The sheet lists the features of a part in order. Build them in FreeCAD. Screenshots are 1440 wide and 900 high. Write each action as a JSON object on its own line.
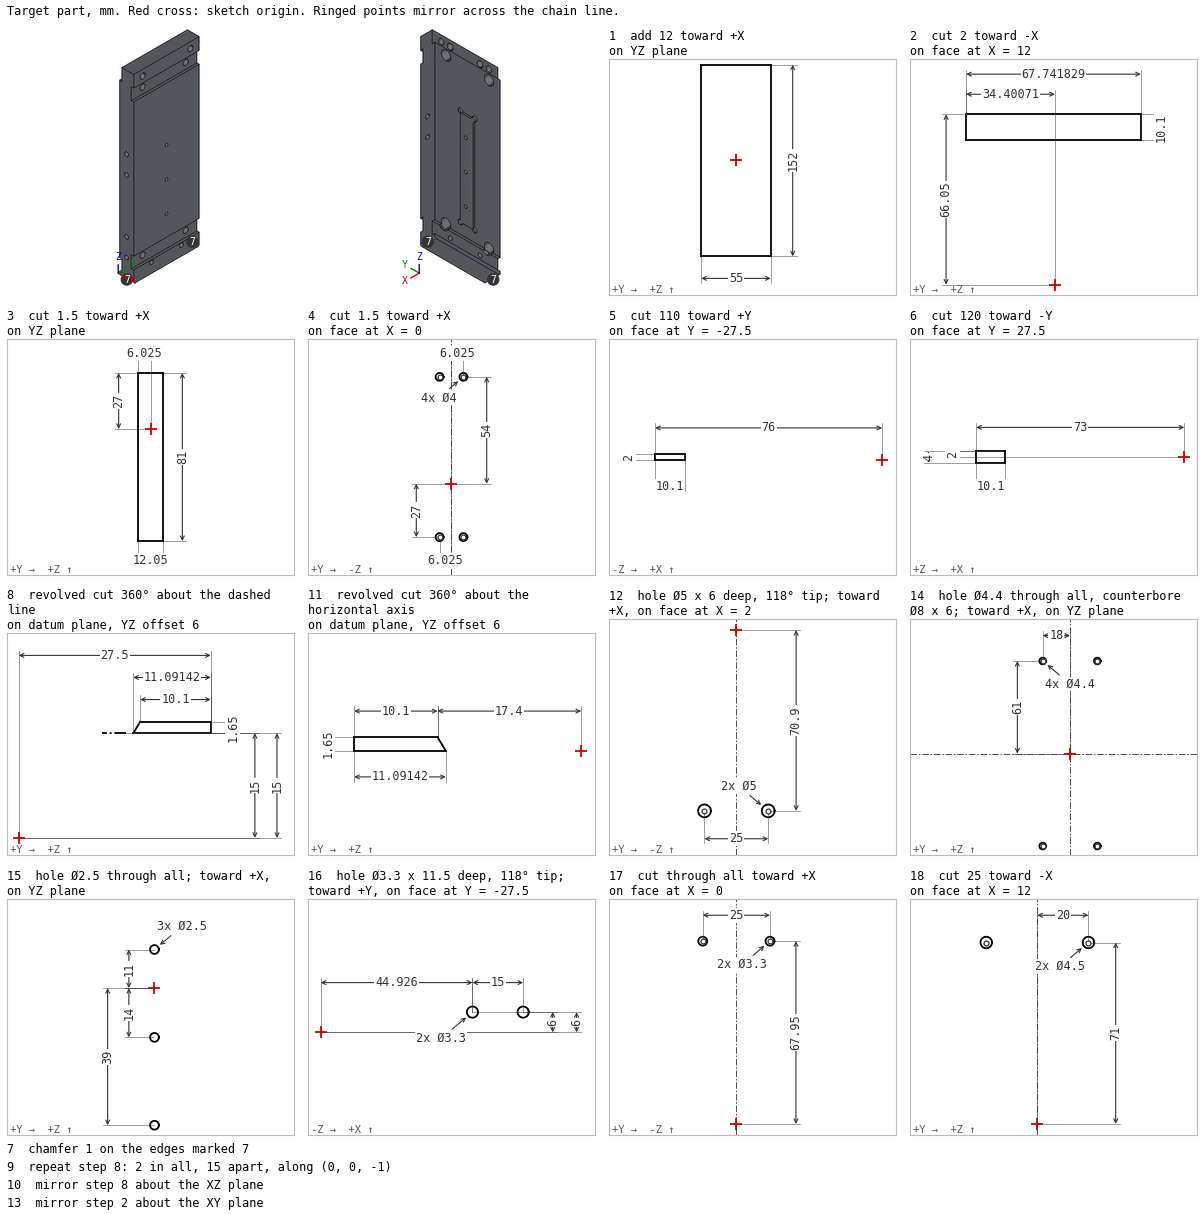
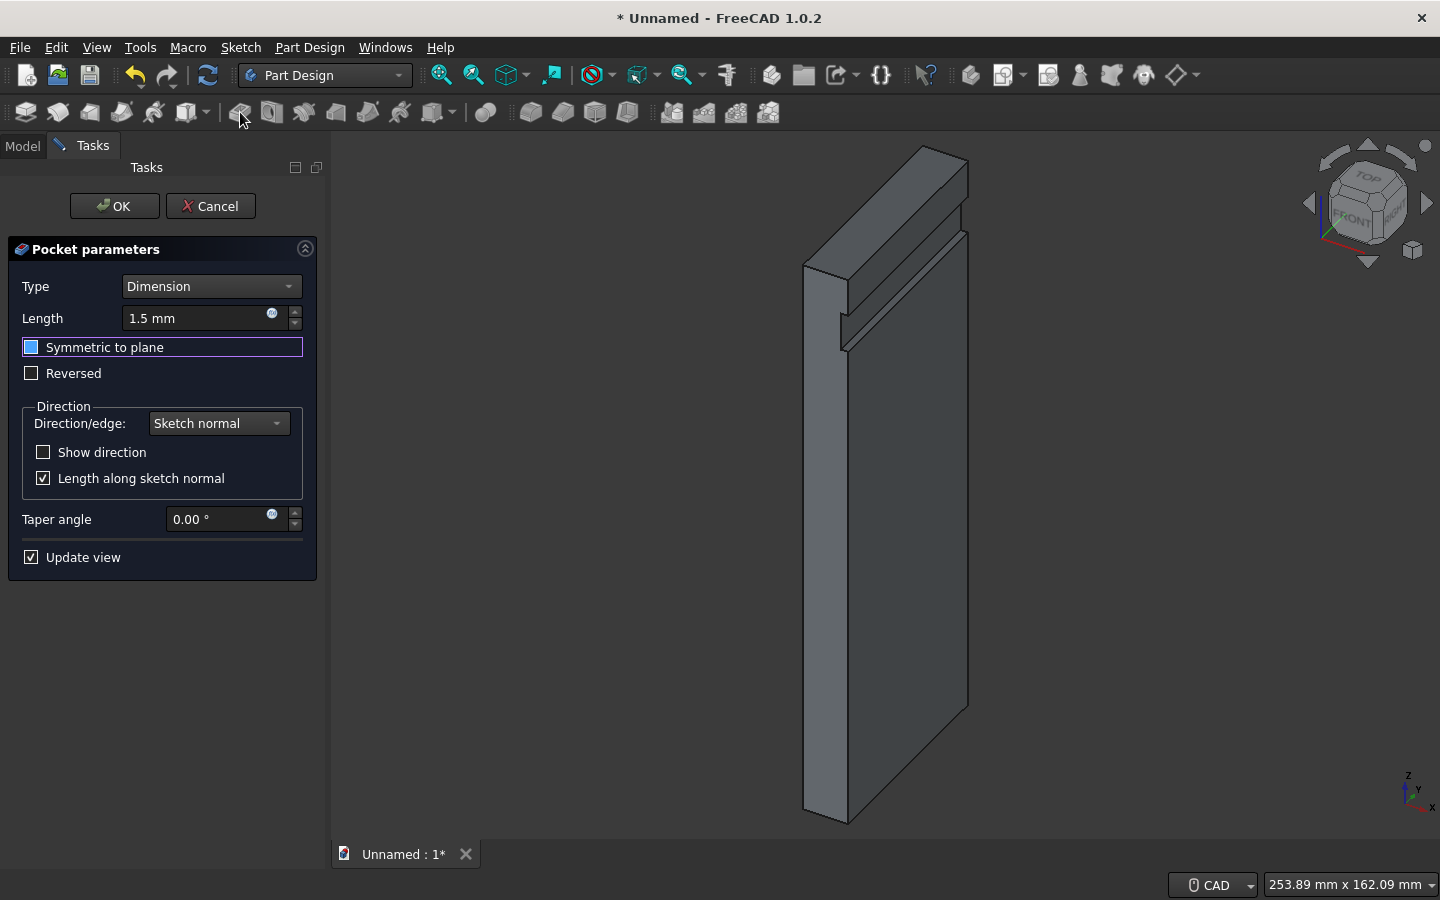
{"action": "left_click", "coordinate": [30, 373]}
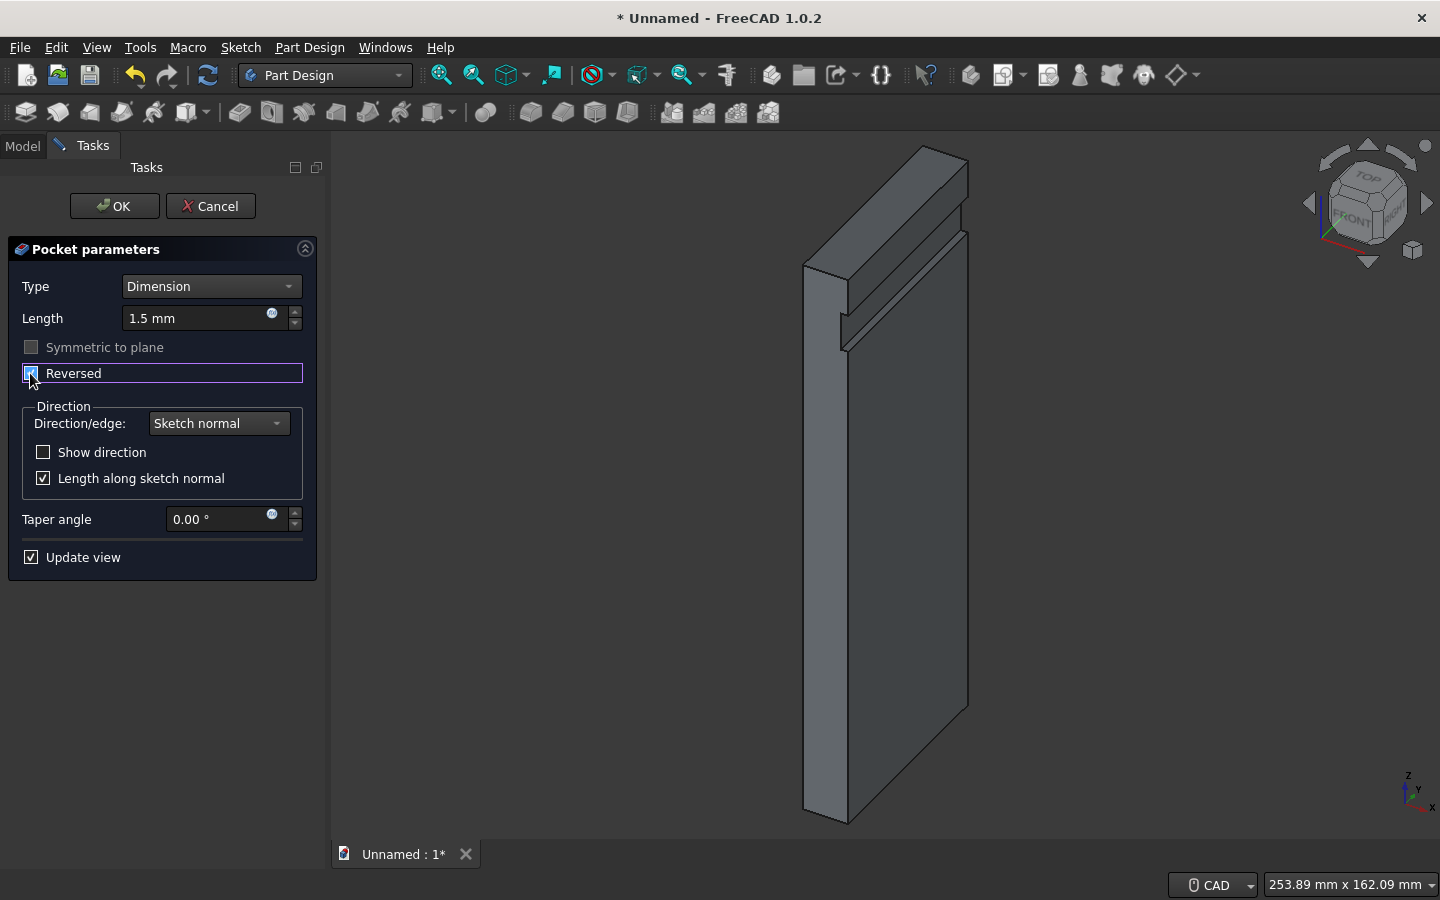
{"action": "left_click", "coordinate": [115, 206]}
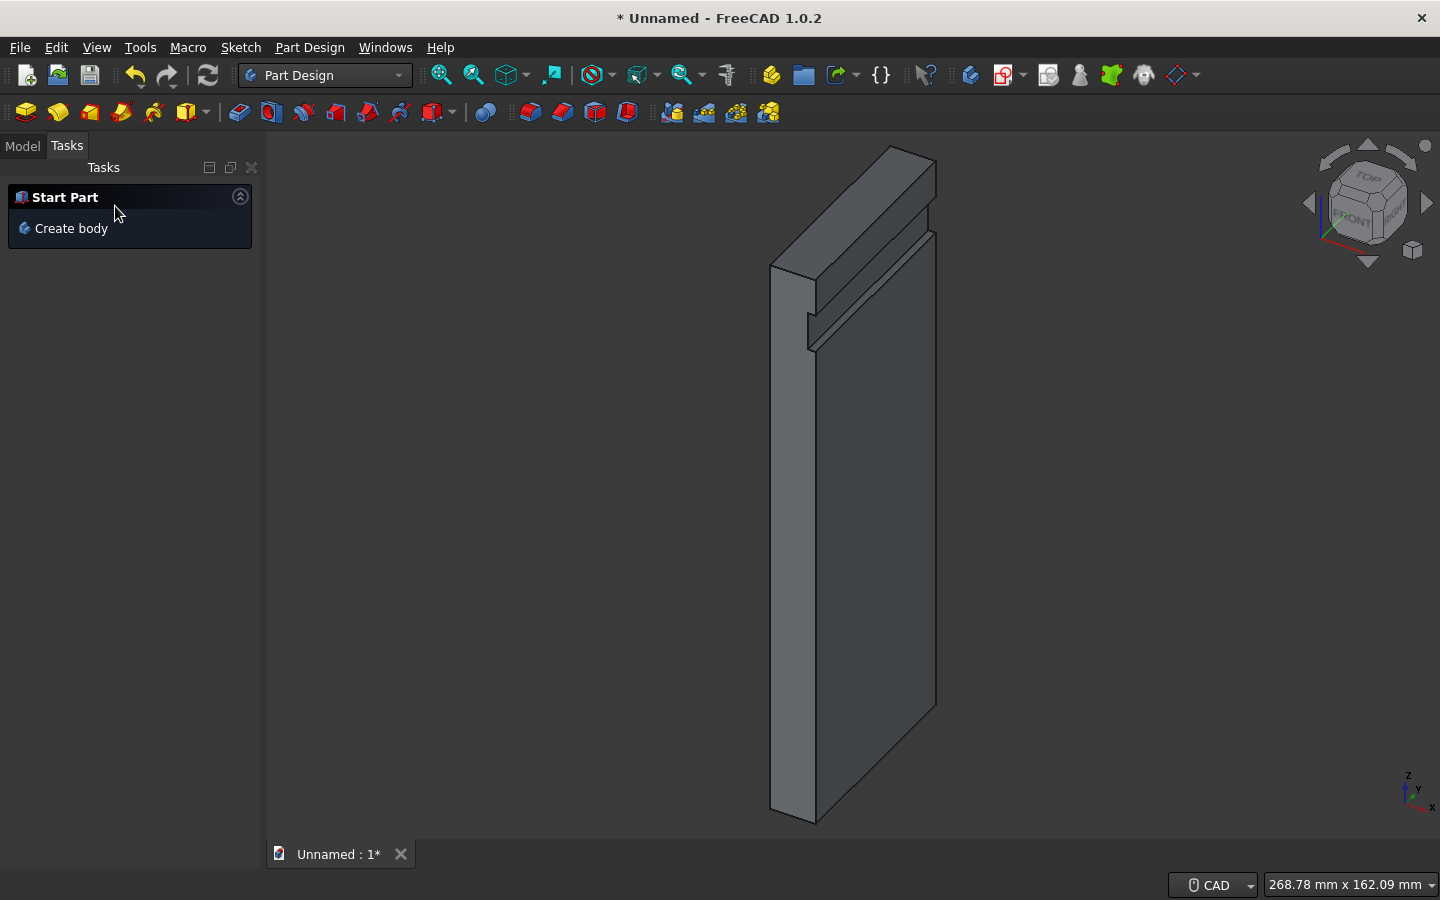
{"action": "key", "text": "6"}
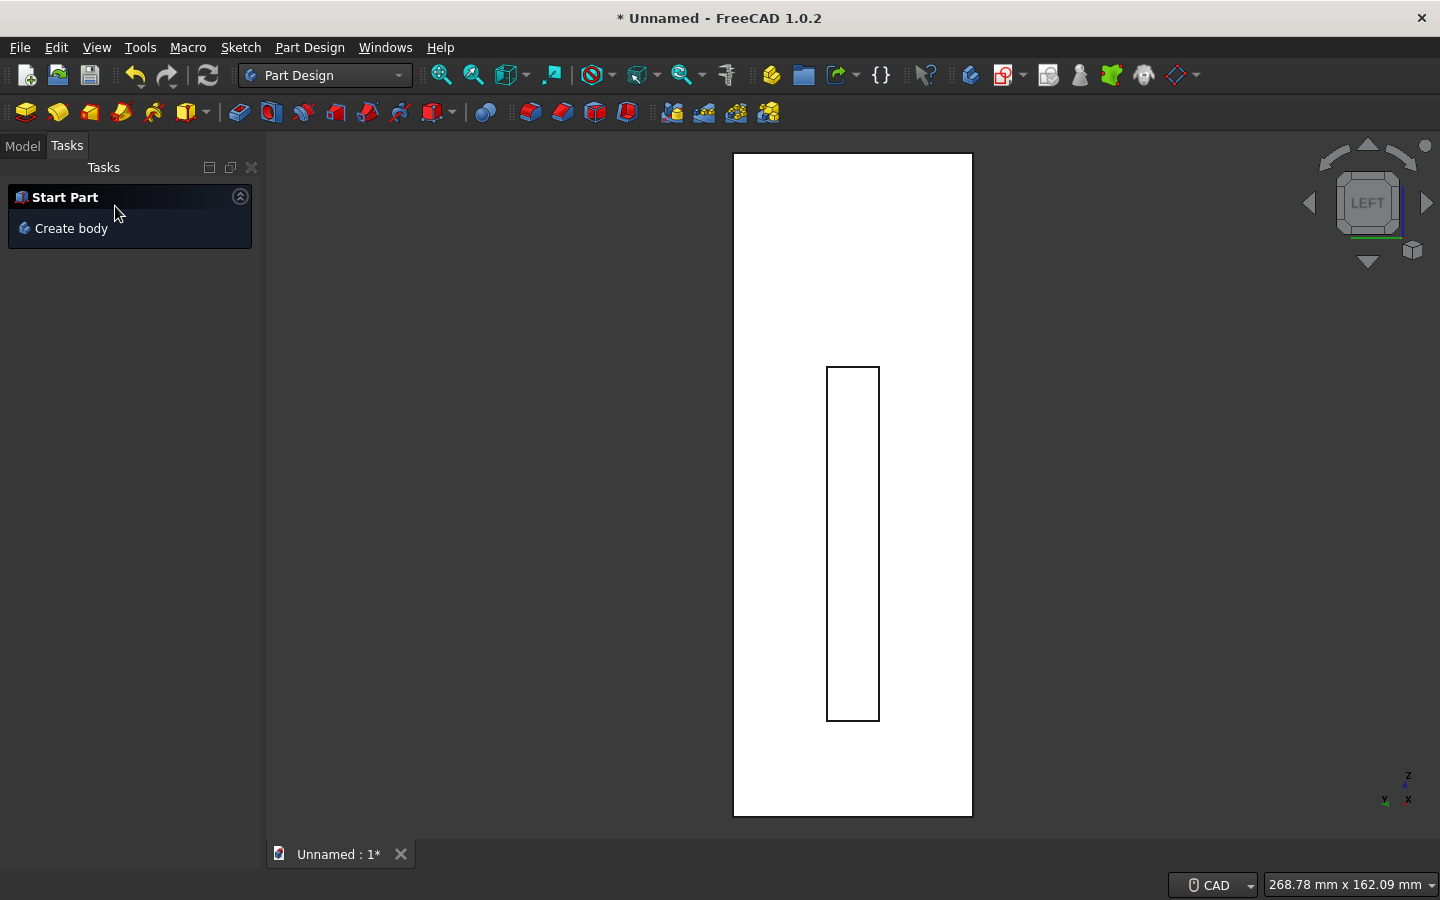
{"action": "left_click", "coordinate": [887, 294]}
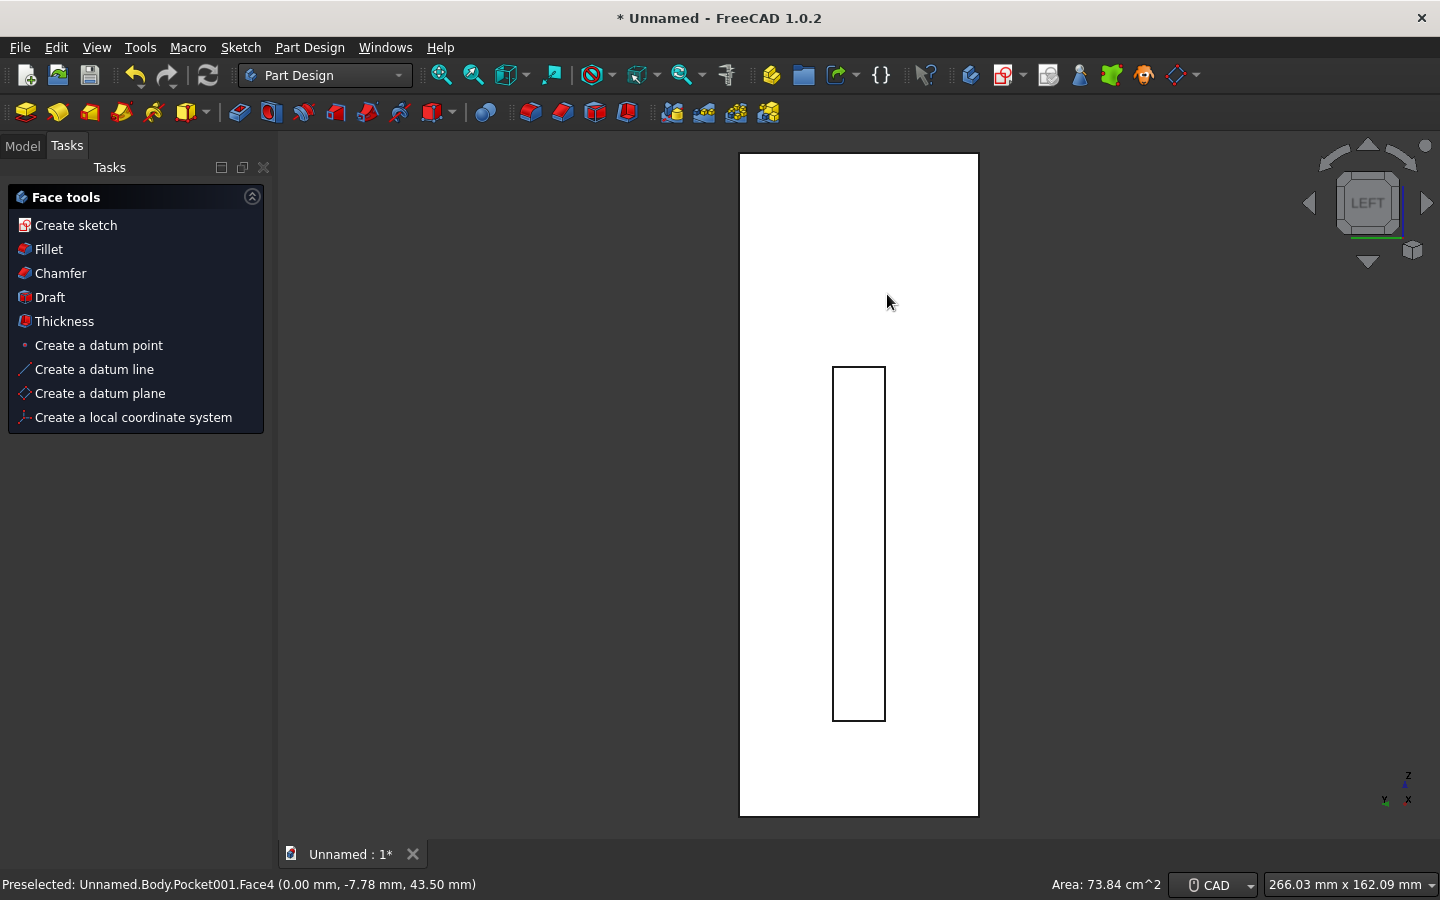
{"action": "left_click", "coordinate": [1004, 76]}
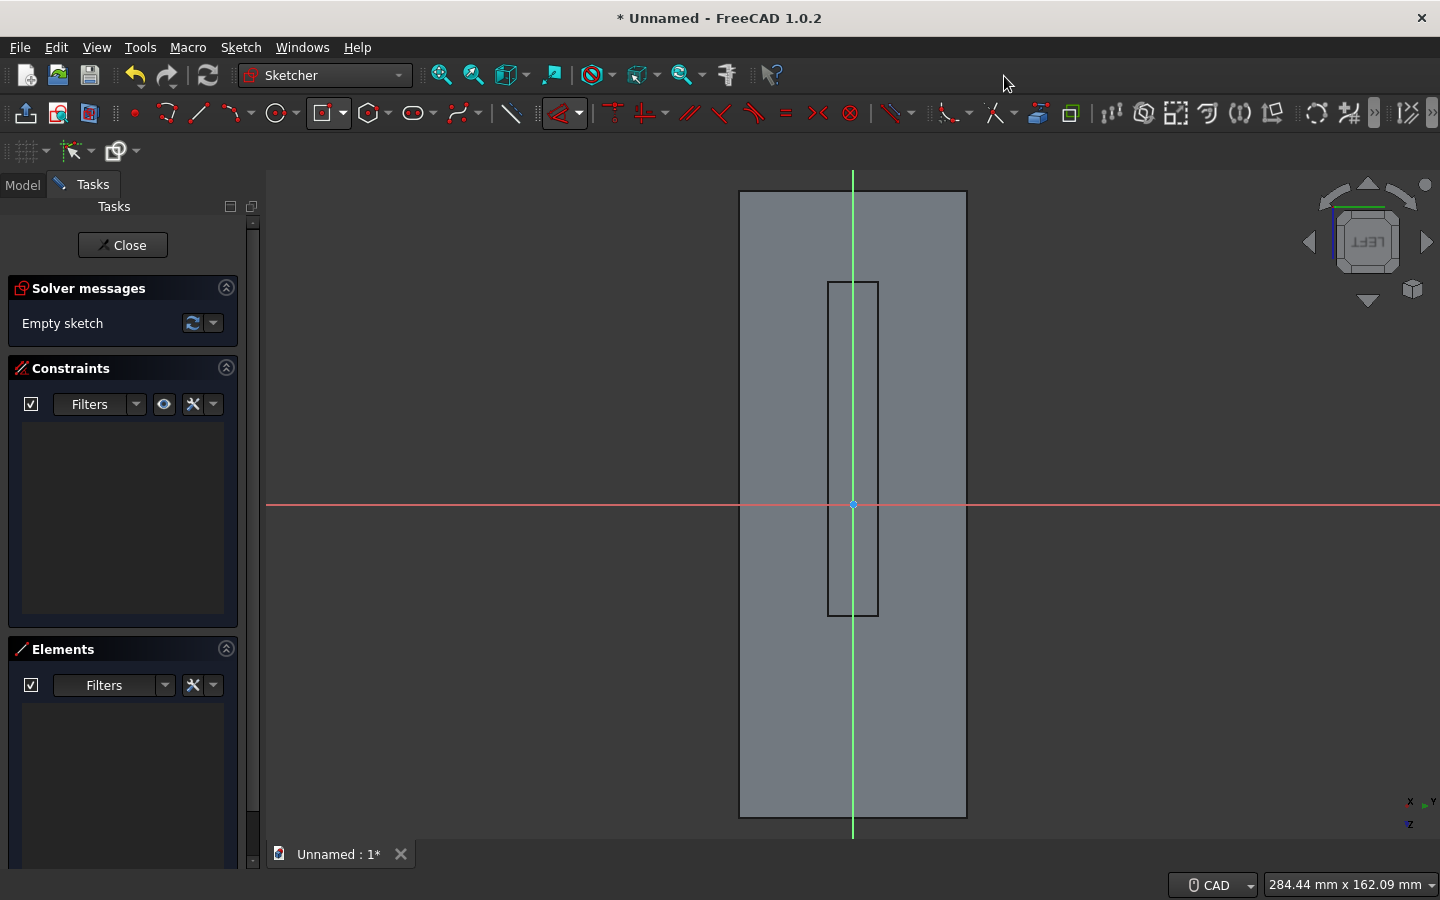
{"action": "left_click", "coordinate": [276, 114]}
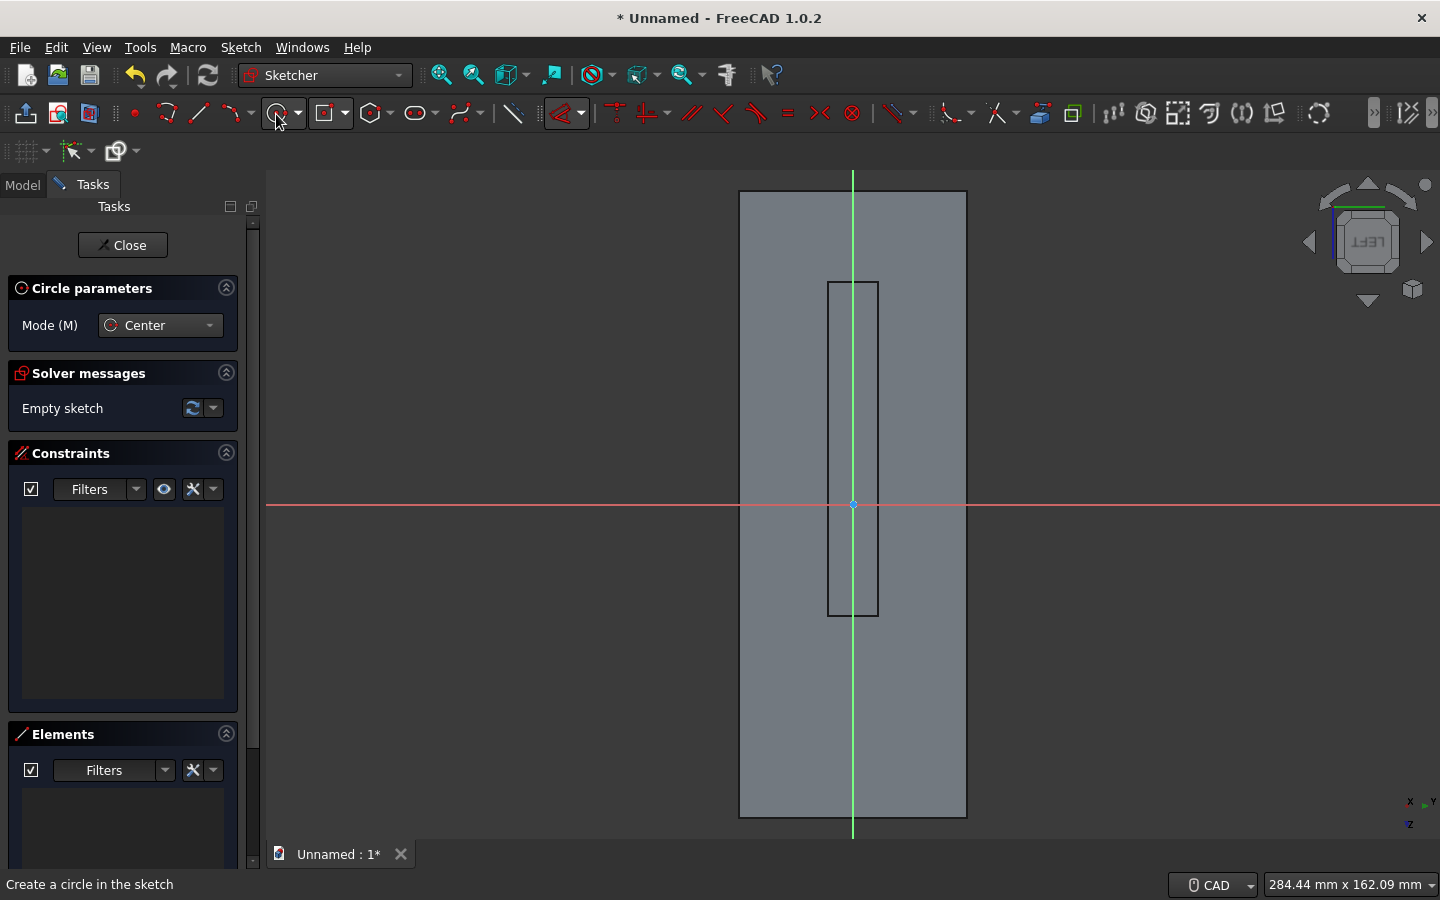
{"action": "scroll", "coordinate": [878, 282], "scroll_direction": "up", "scroll_amount": 6}